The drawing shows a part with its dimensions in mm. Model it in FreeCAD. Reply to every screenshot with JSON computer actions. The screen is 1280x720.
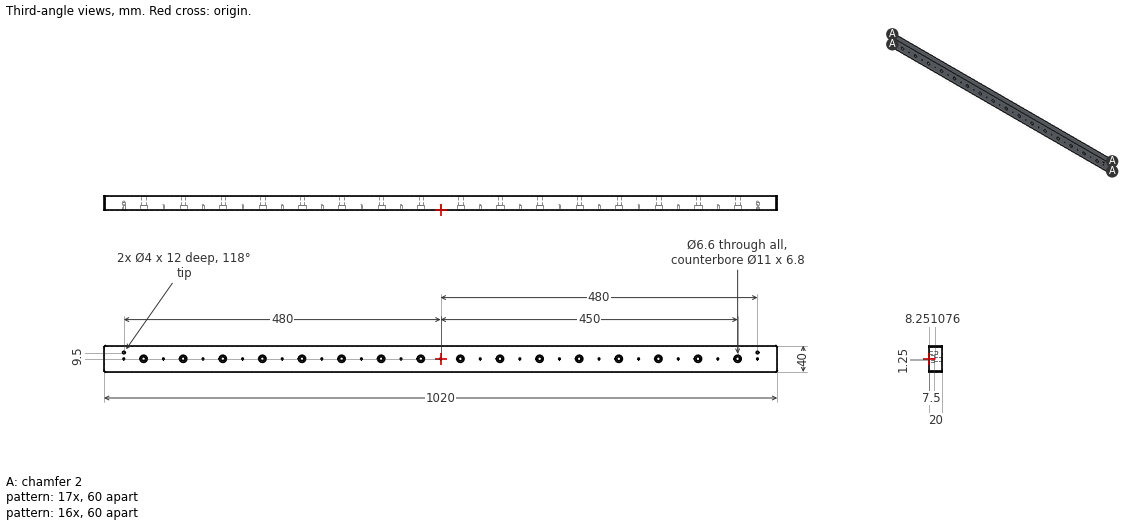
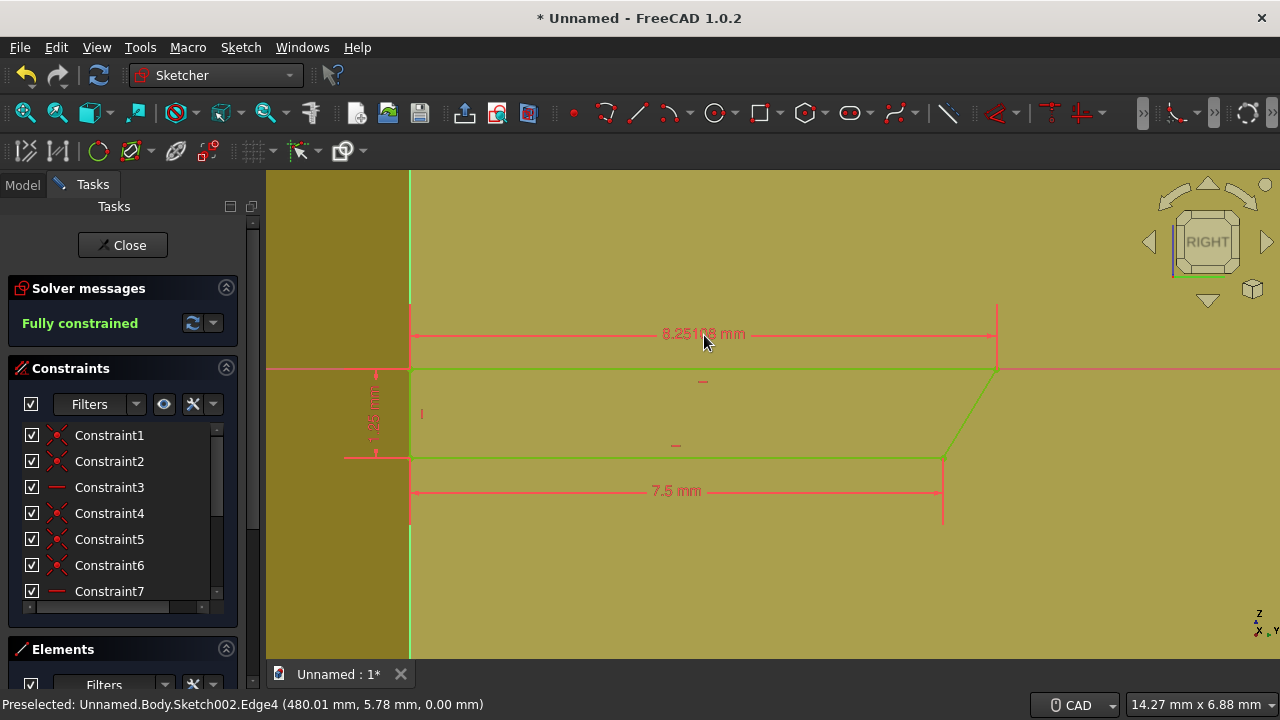
{"action": "left_click", "coordinate": [123, 245]}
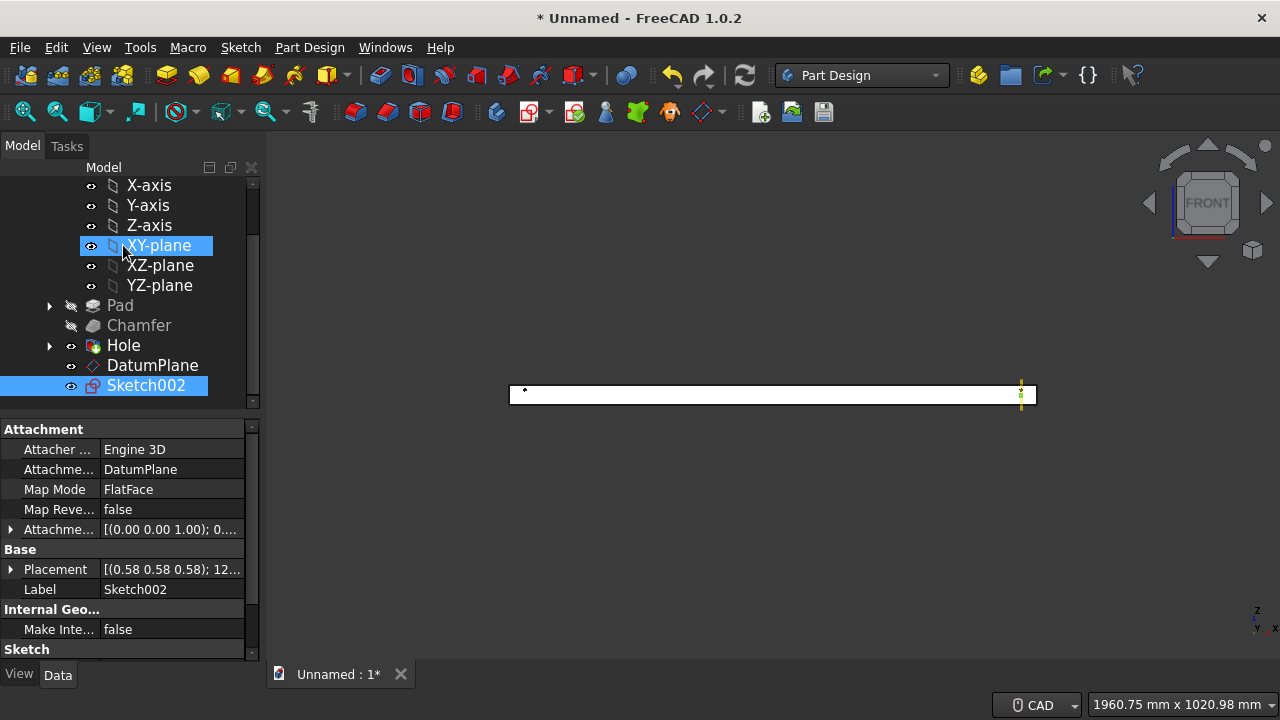
{"action": "left_click", "coordinate": [446, 76]}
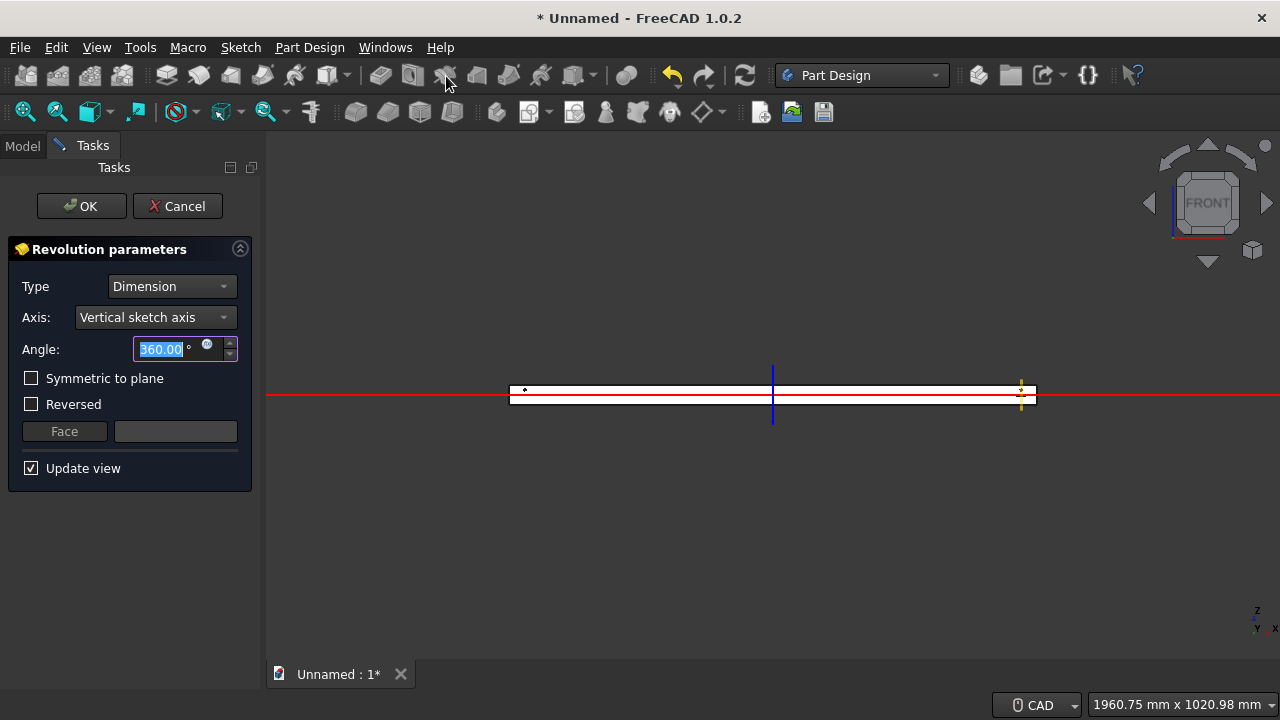
{"action": "left_click", "coordinate": [156, 318]}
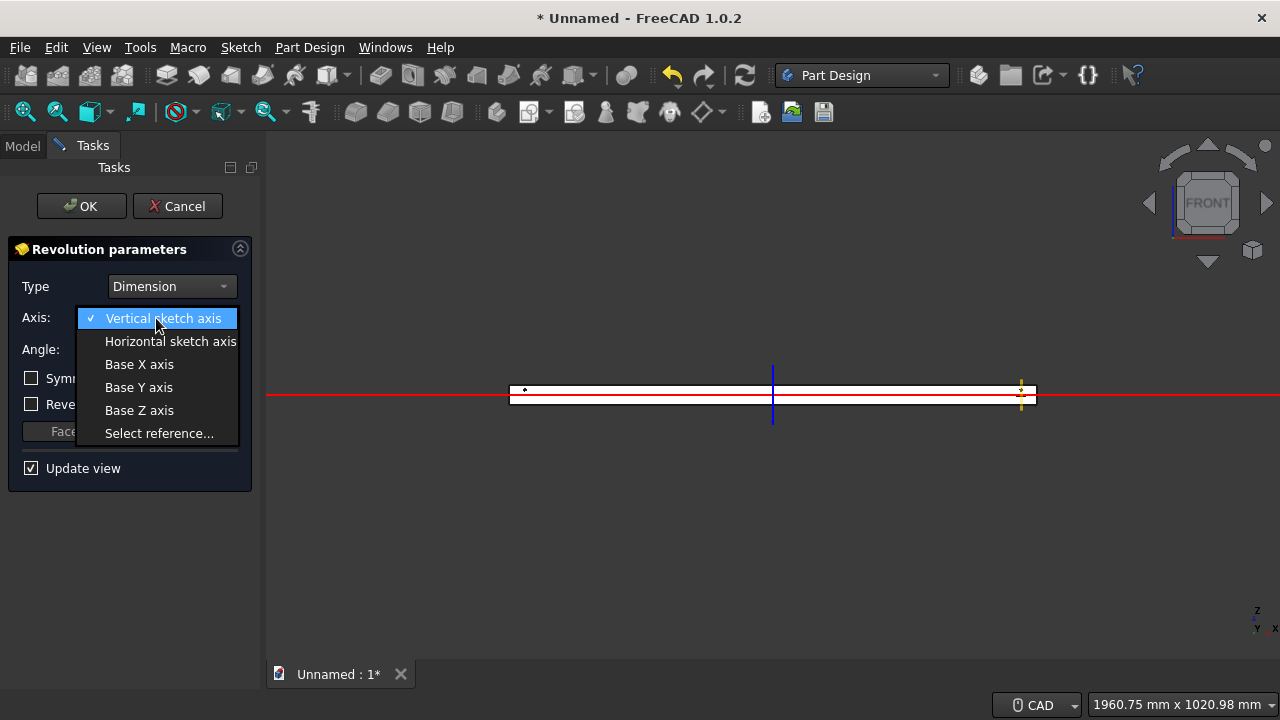
{"action": "left_click", "coordinate": [156, 342]}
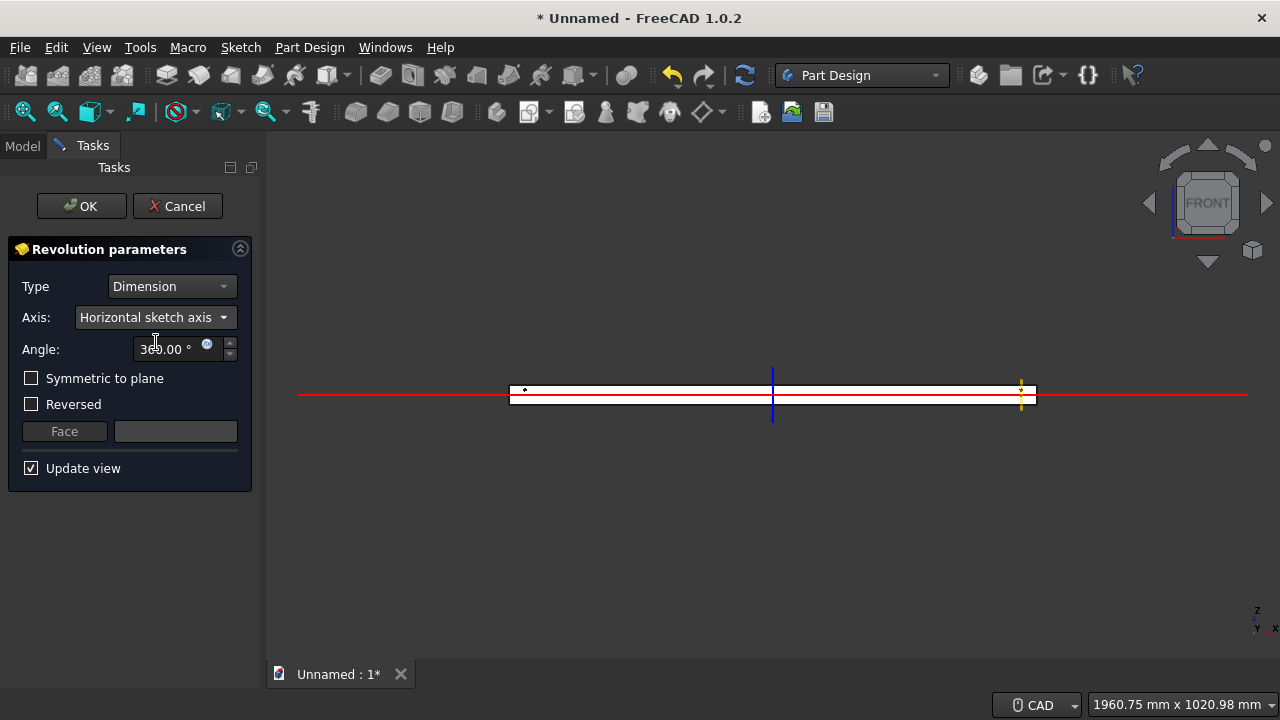
{"action": "left_click", "coordinate": [82, 206]}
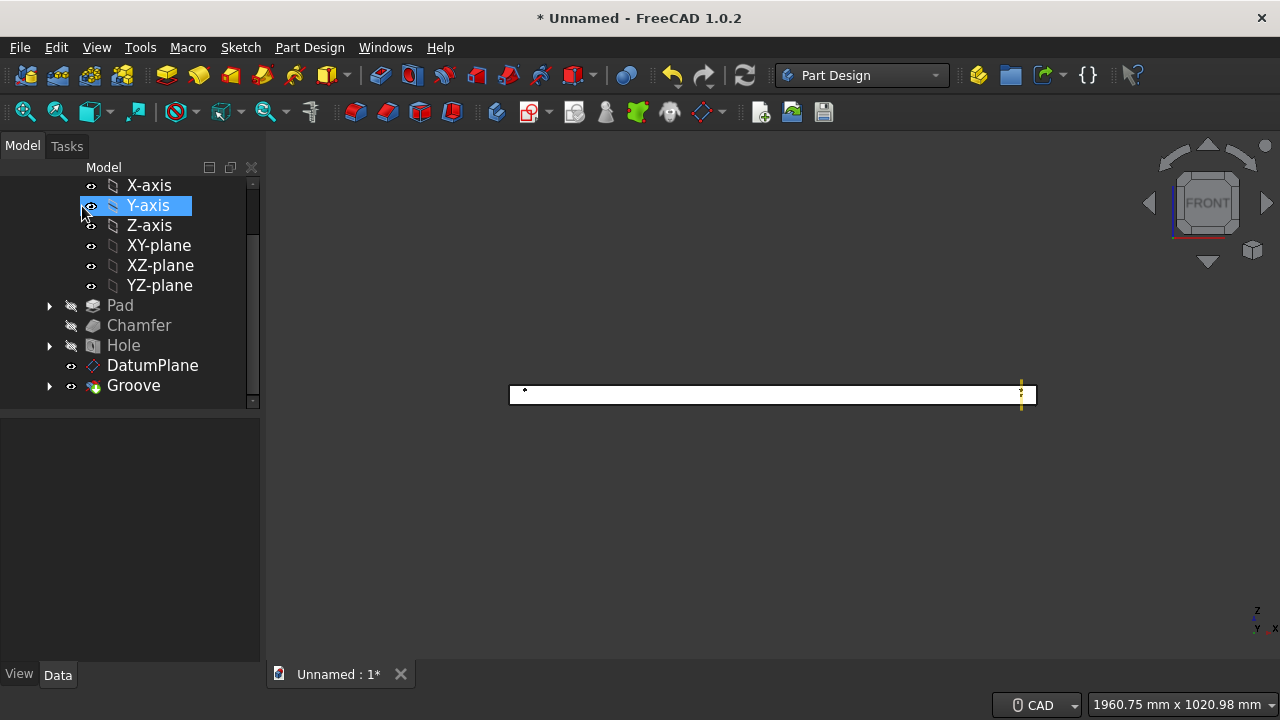
{"action": "left_click", "coordinate": [116, 366]}
{"action": "key", "text": "space"}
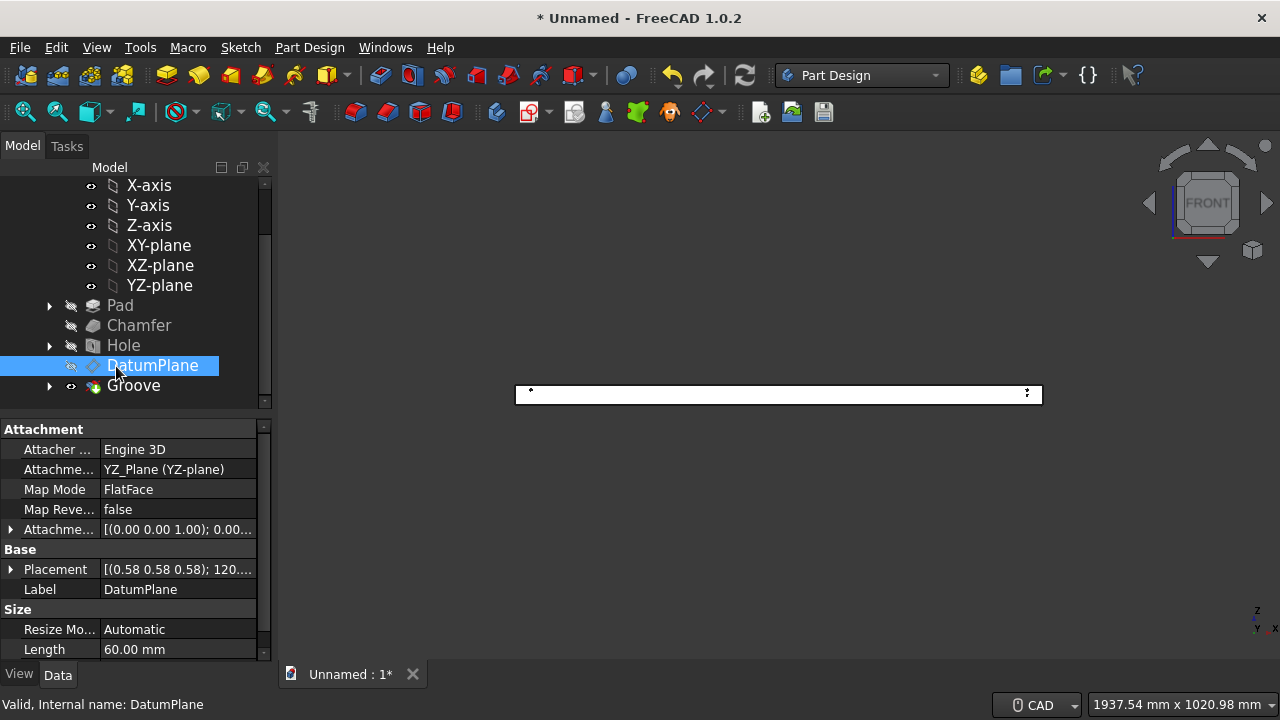
{"action": "left_click", "coordinate": [116, 386]}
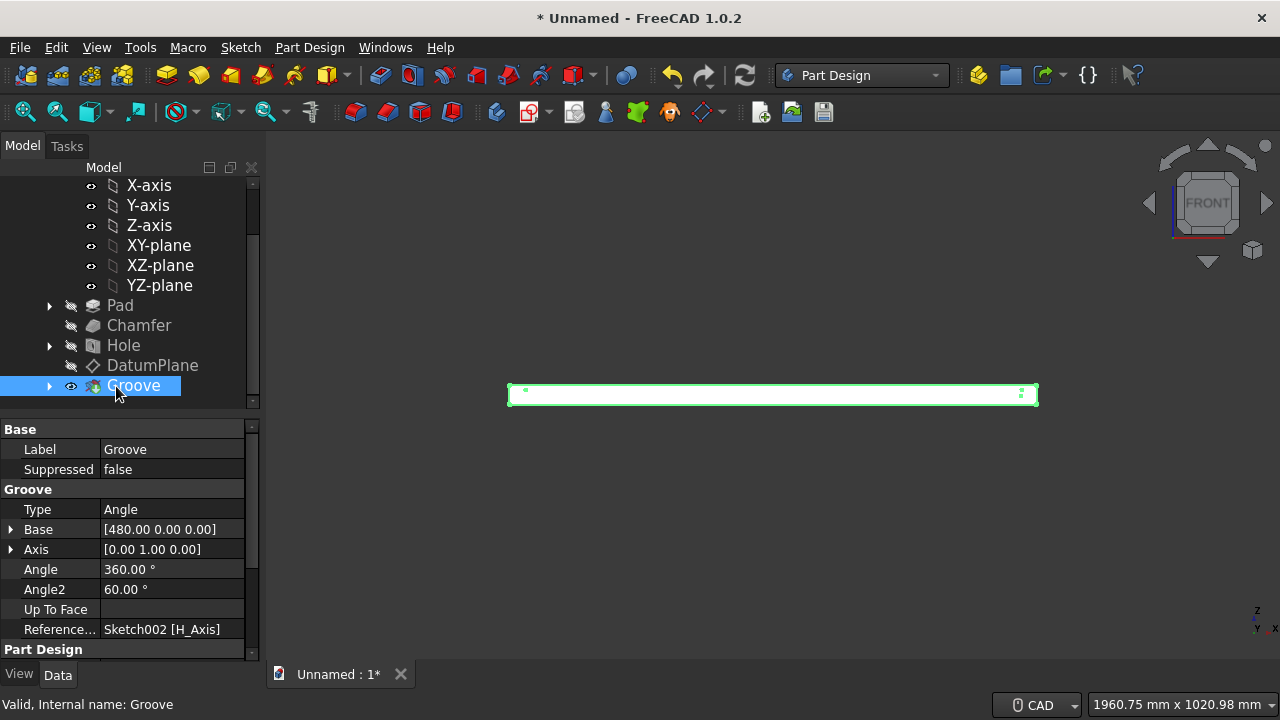
{"action": "left_click", "coordinate": [58, 76]}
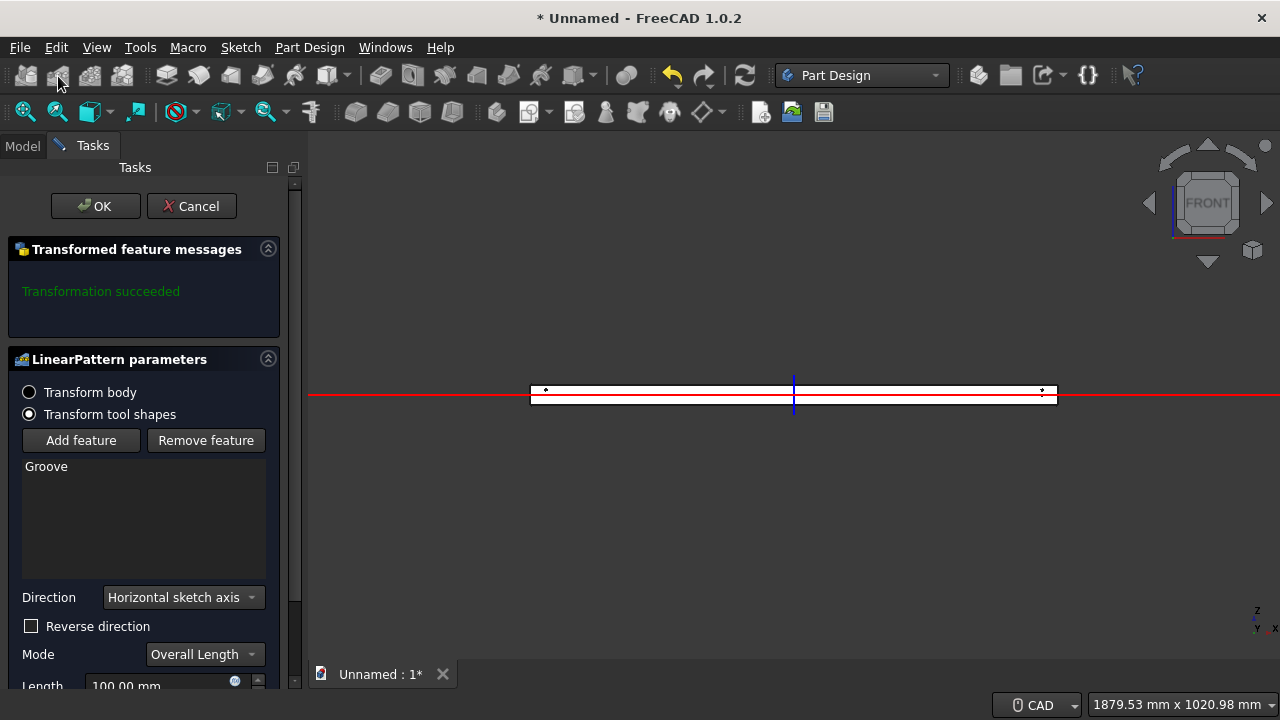
{"action": "left_click", "coordinate": [184, 598]}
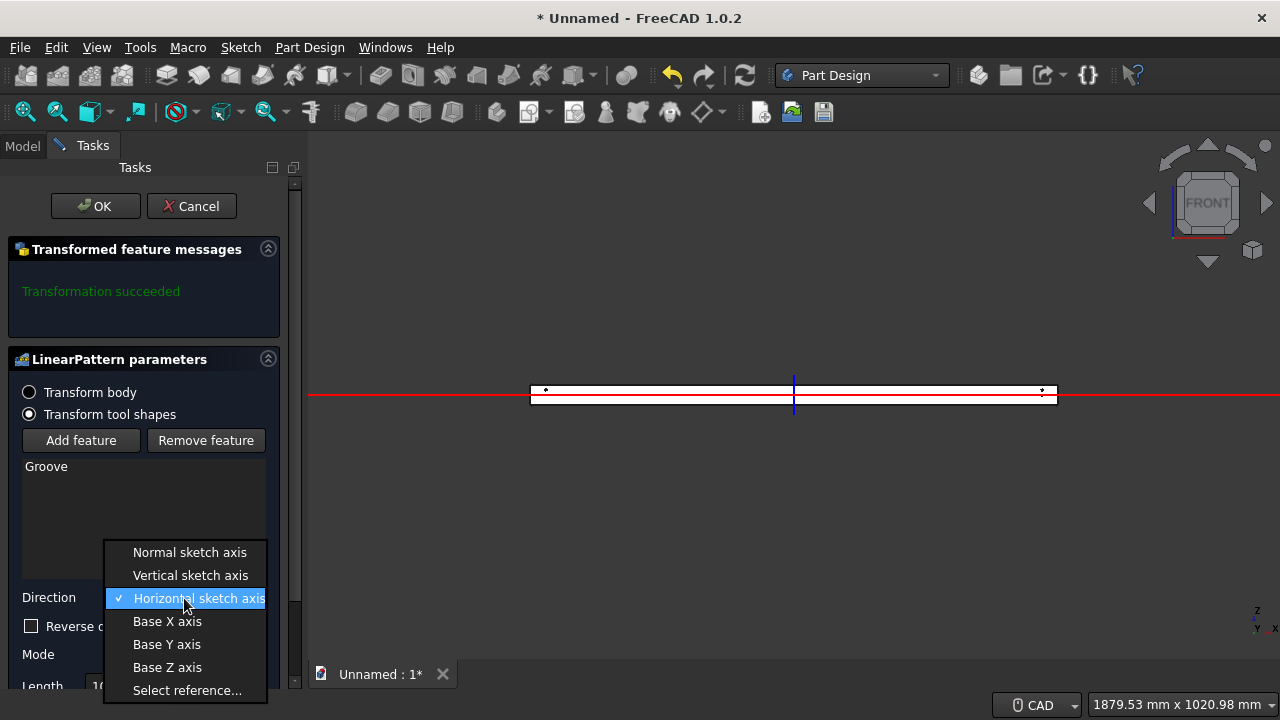
{"action": "left_click", "coordinate": [184, 622]}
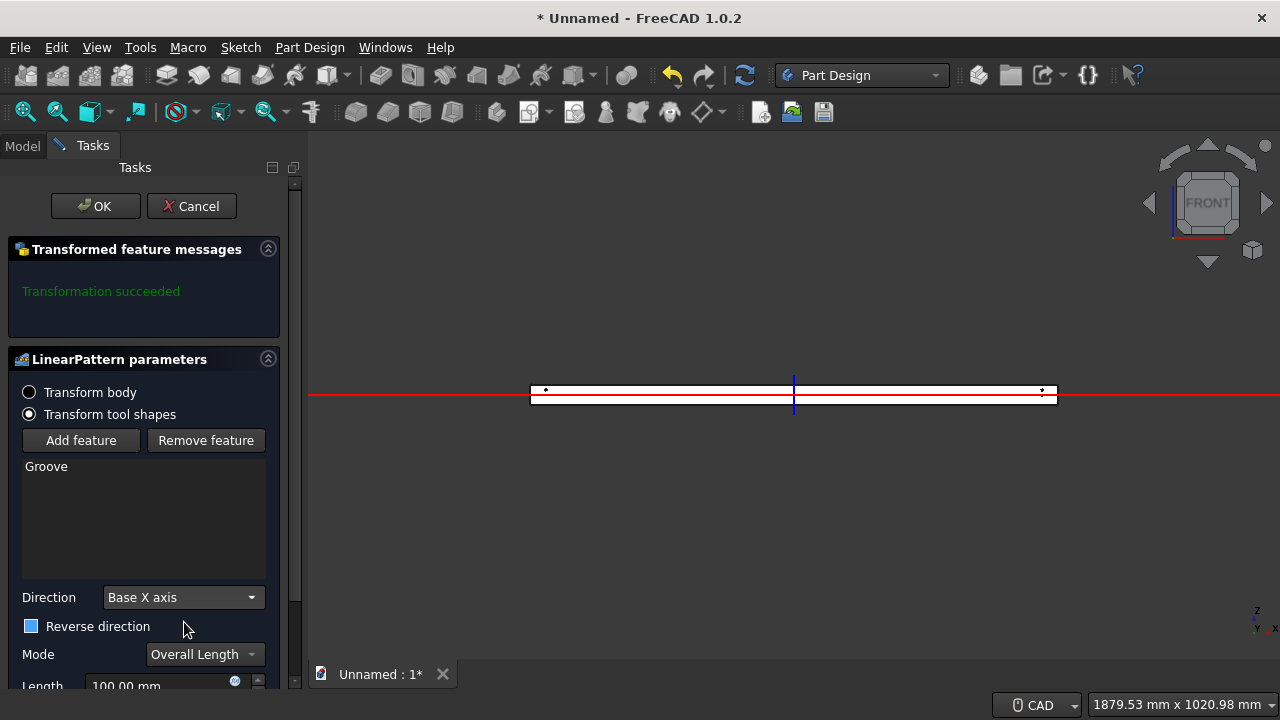
{"action": "left_click", "coordinate": [206, 654]}